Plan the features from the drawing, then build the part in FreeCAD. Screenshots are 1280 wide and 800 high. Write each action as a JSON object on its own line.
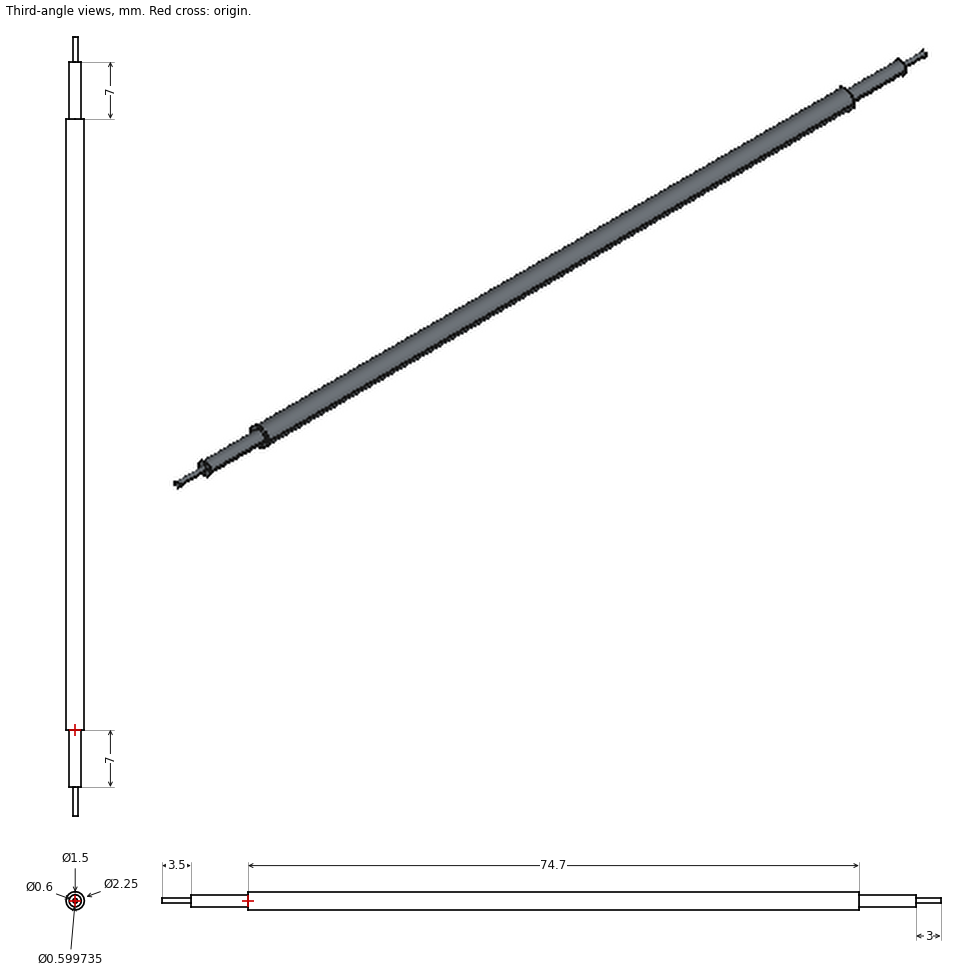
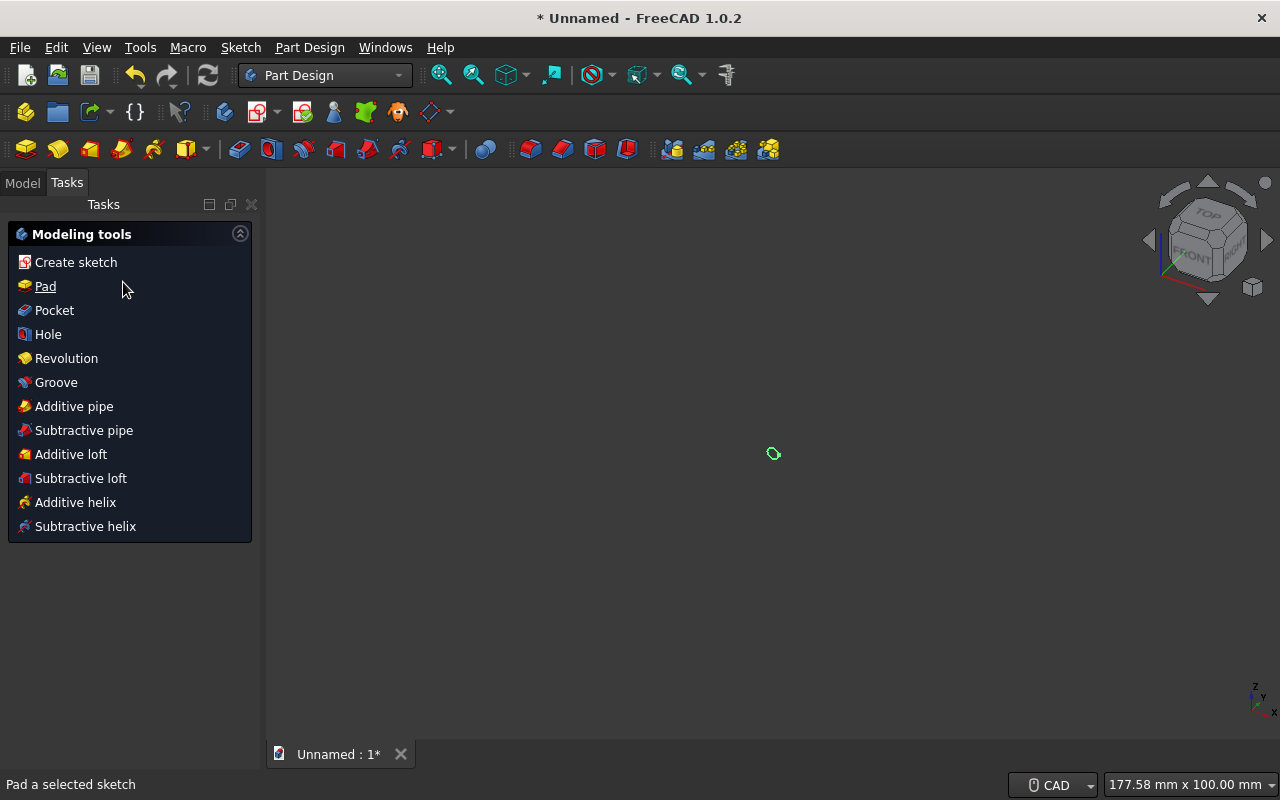
{"action": "left_click", "coordinate": [26, 150]}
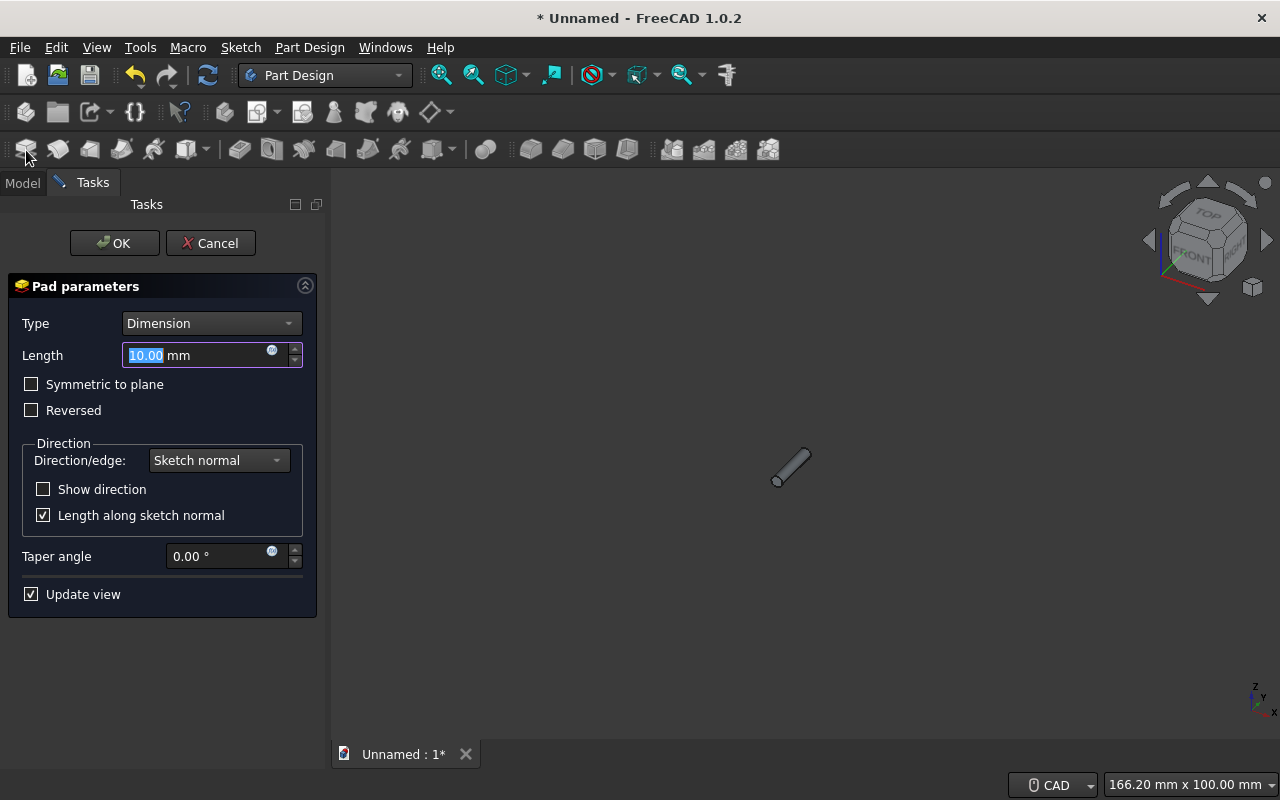
{"action": "type", "text": "74.7"}
{"action": "key", "text": "Tab"}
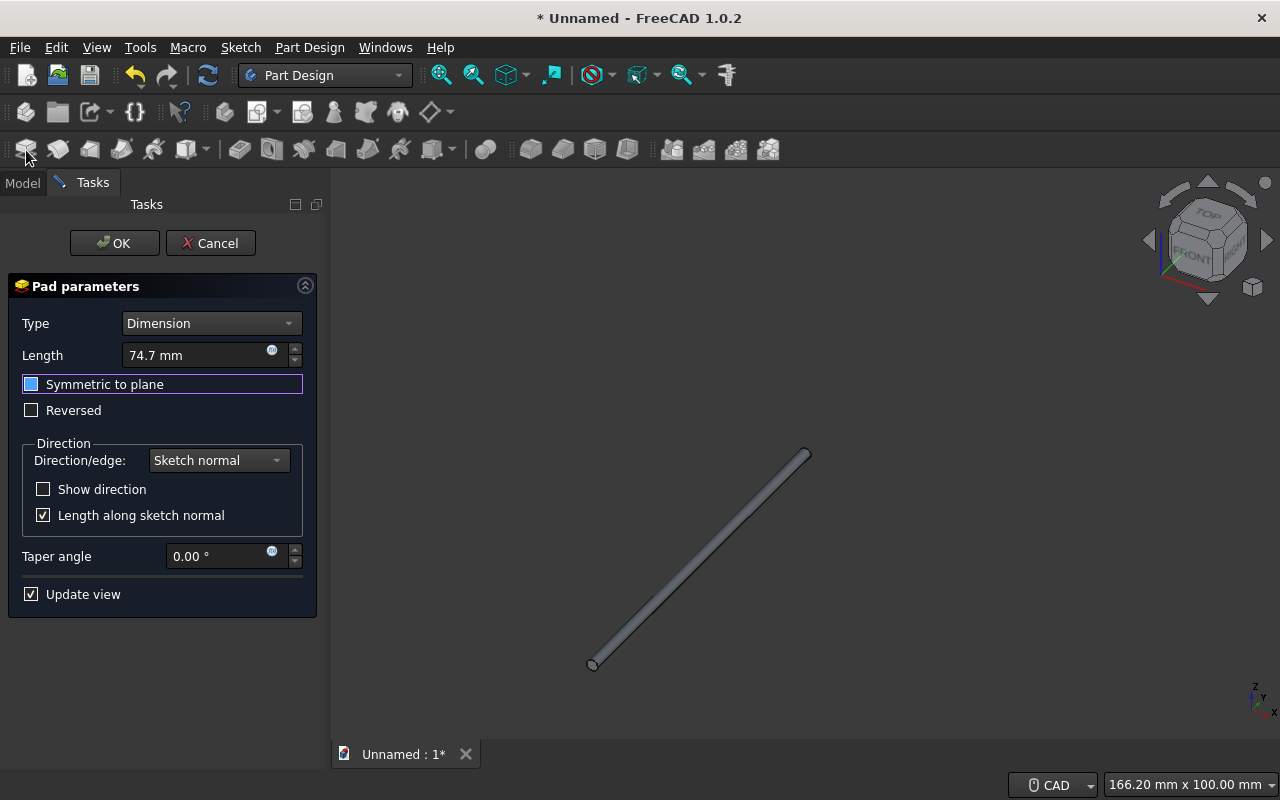
{"action": "left_click", "coordinate": [30, 410]}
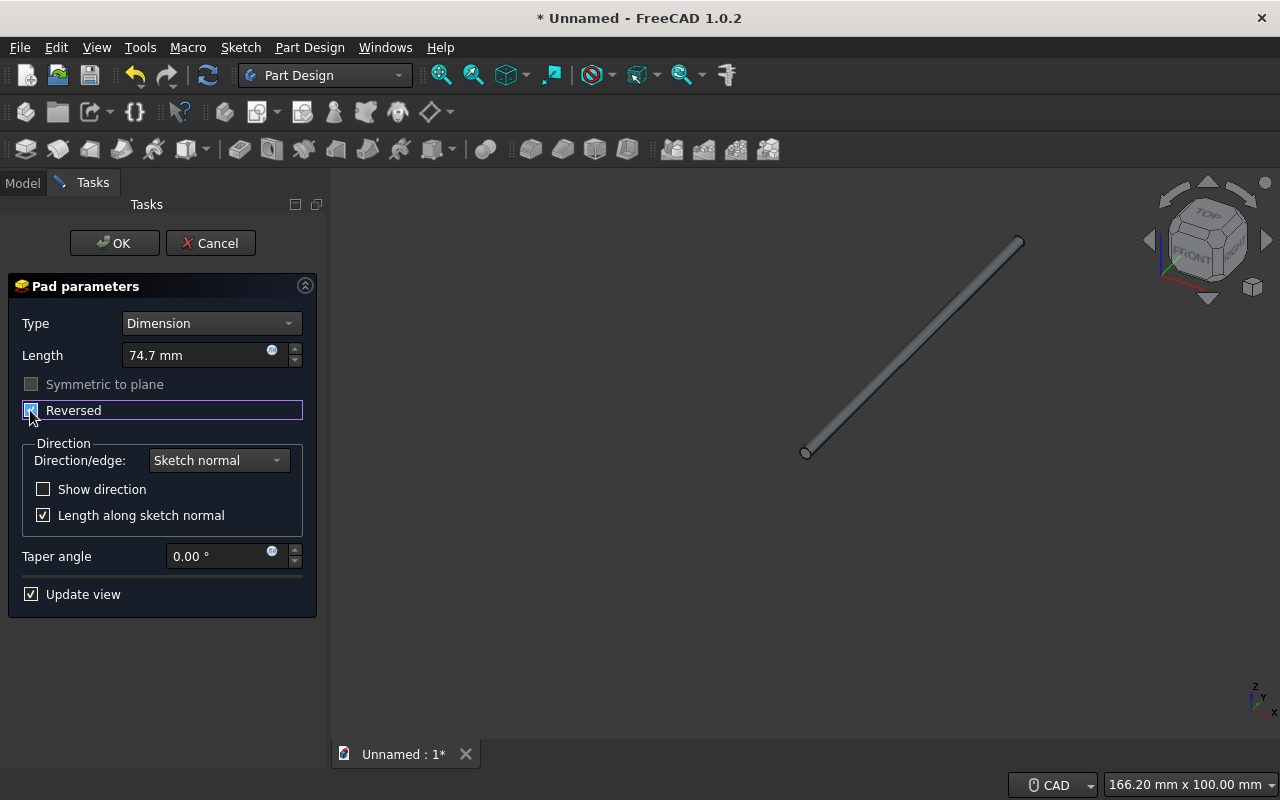
{"action": "left_click", "coordinate": [115, 243]}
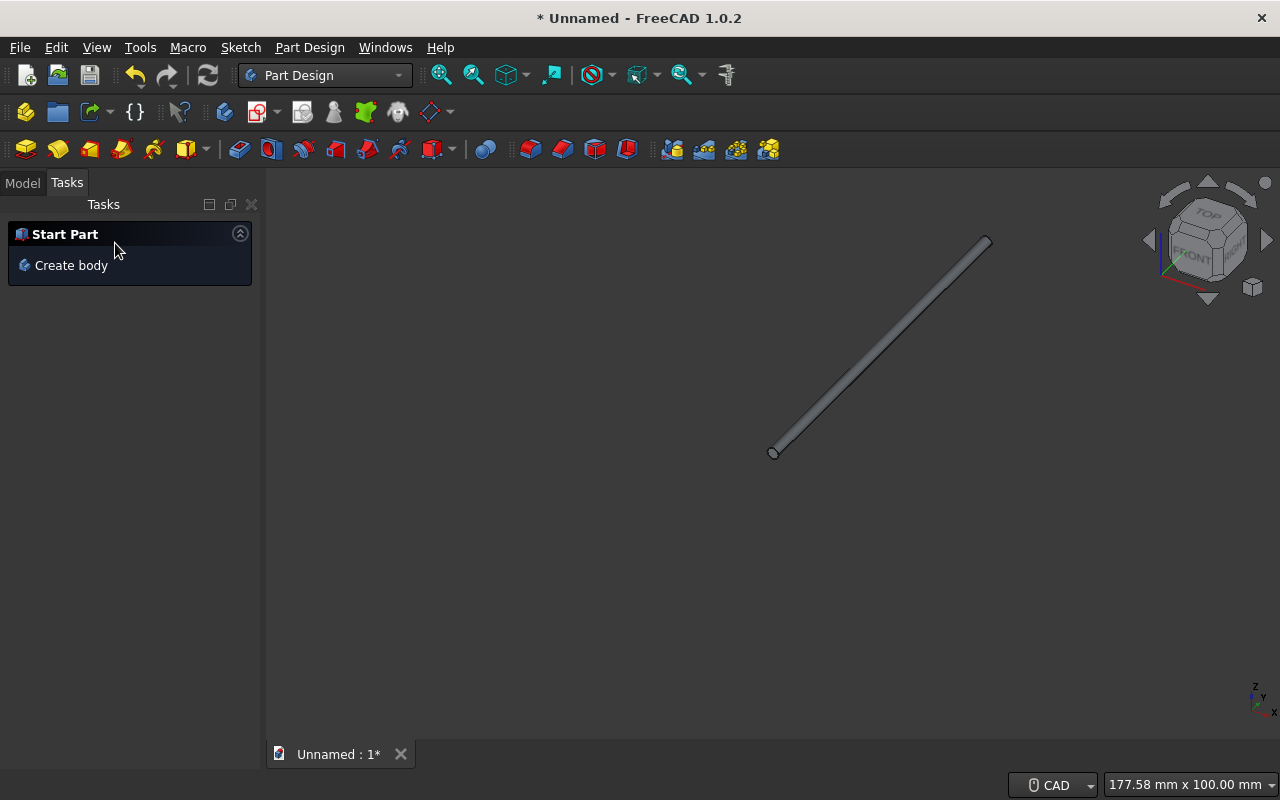
{"action": "left_click", "coordinate": [442, 76]}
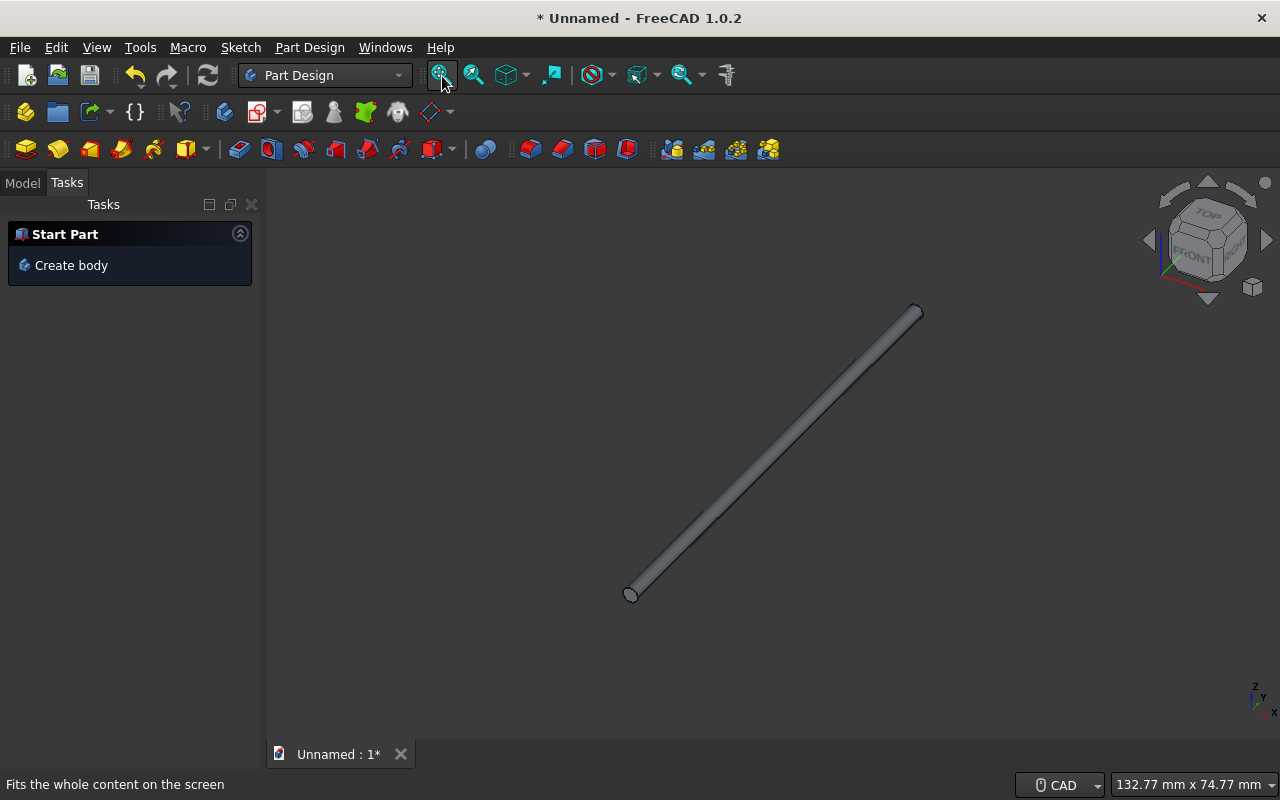
{"action": "left_click", "coordinate": [258, 112]}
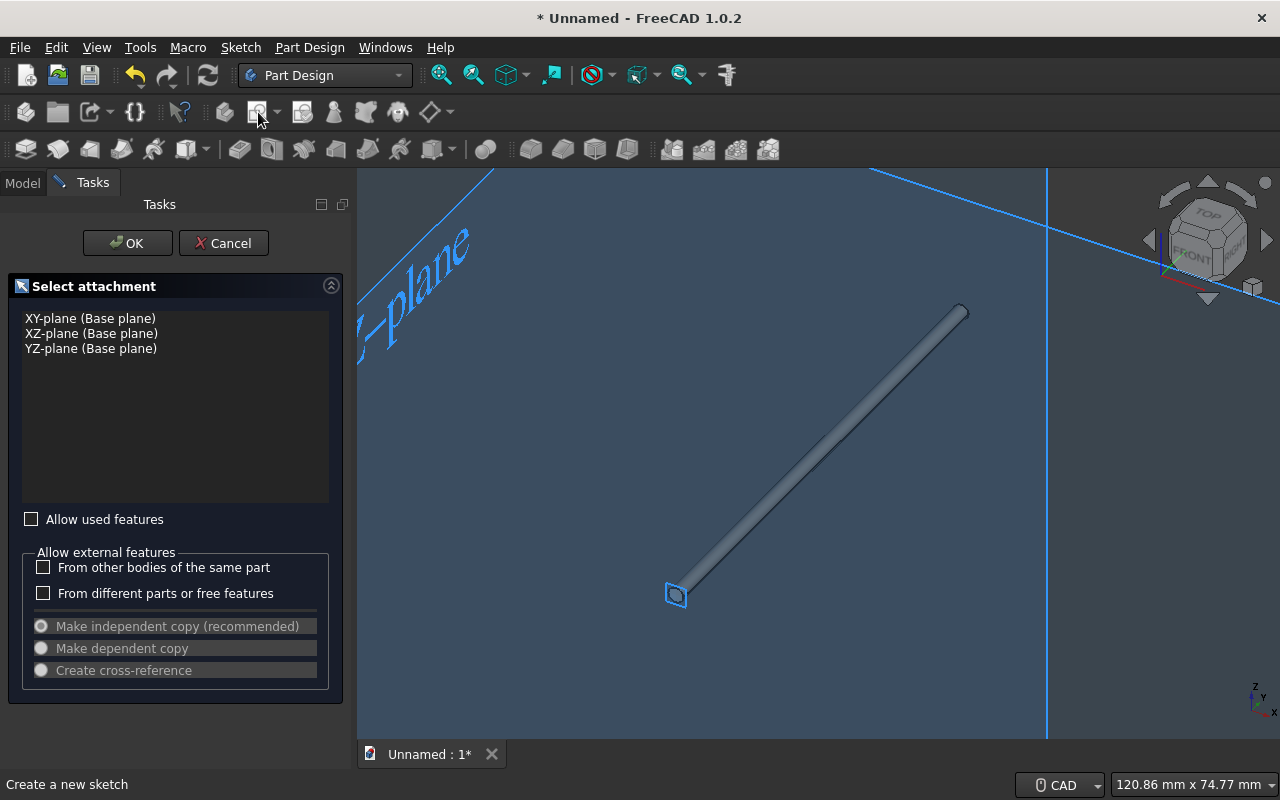
{"action": "left_click", "coordinate": [82, 334]}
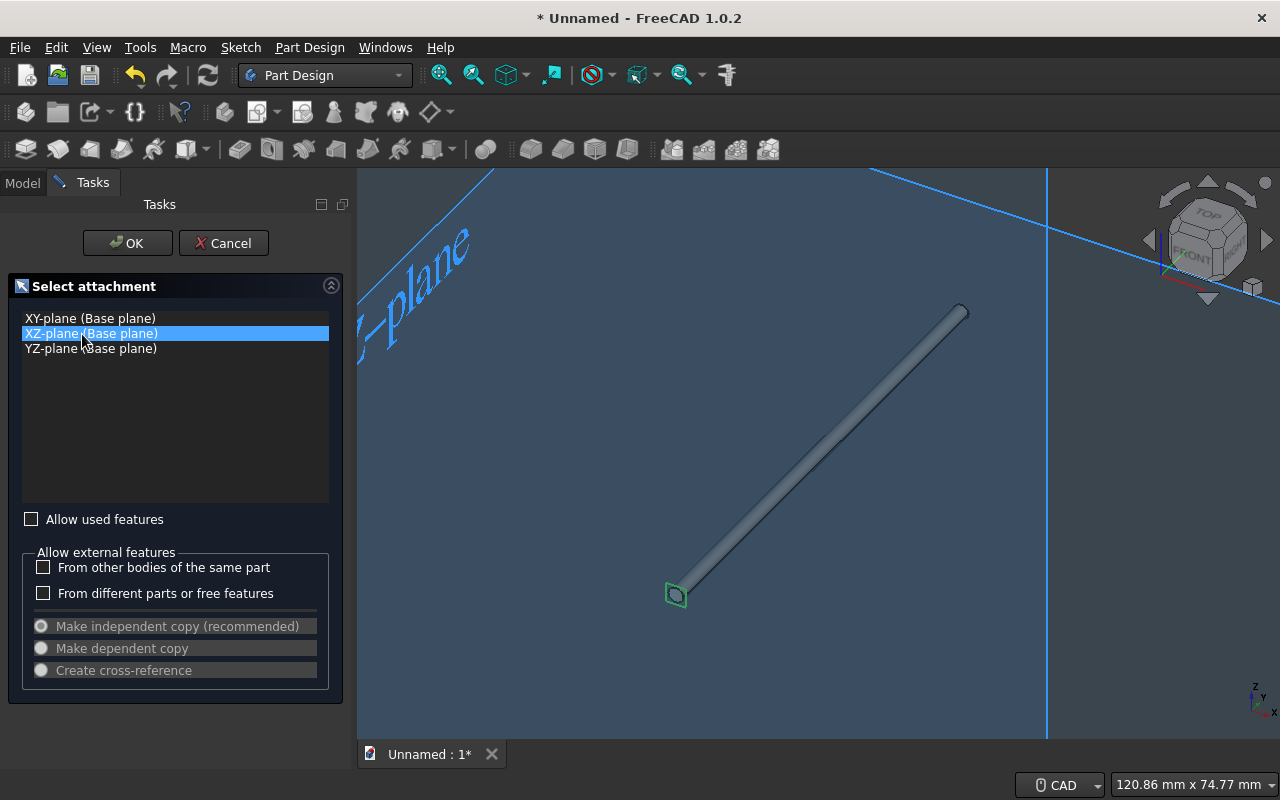
{"action": "left_click", "coordinate": [128, 243]}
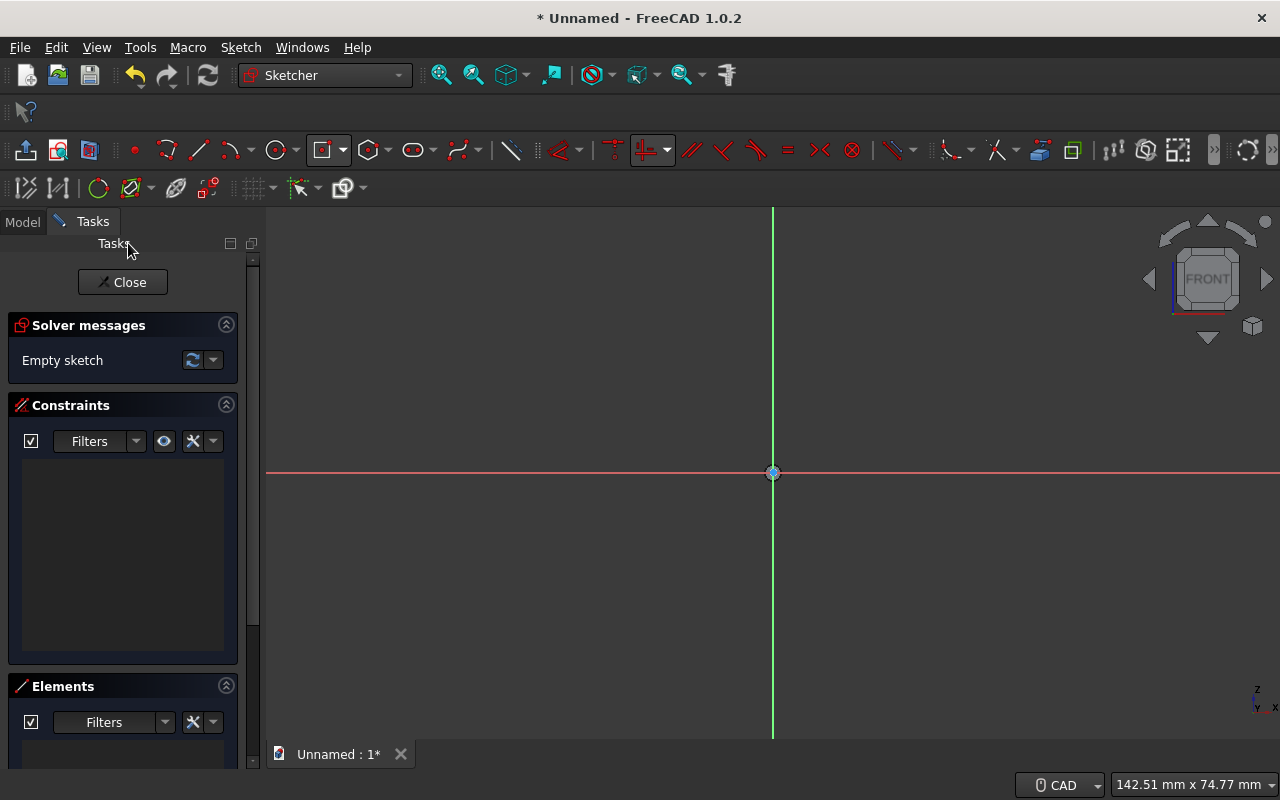
{"action": "scroll", "coordinate": [777, 473], "scroll_direction": "up", "scroll_amount": 15}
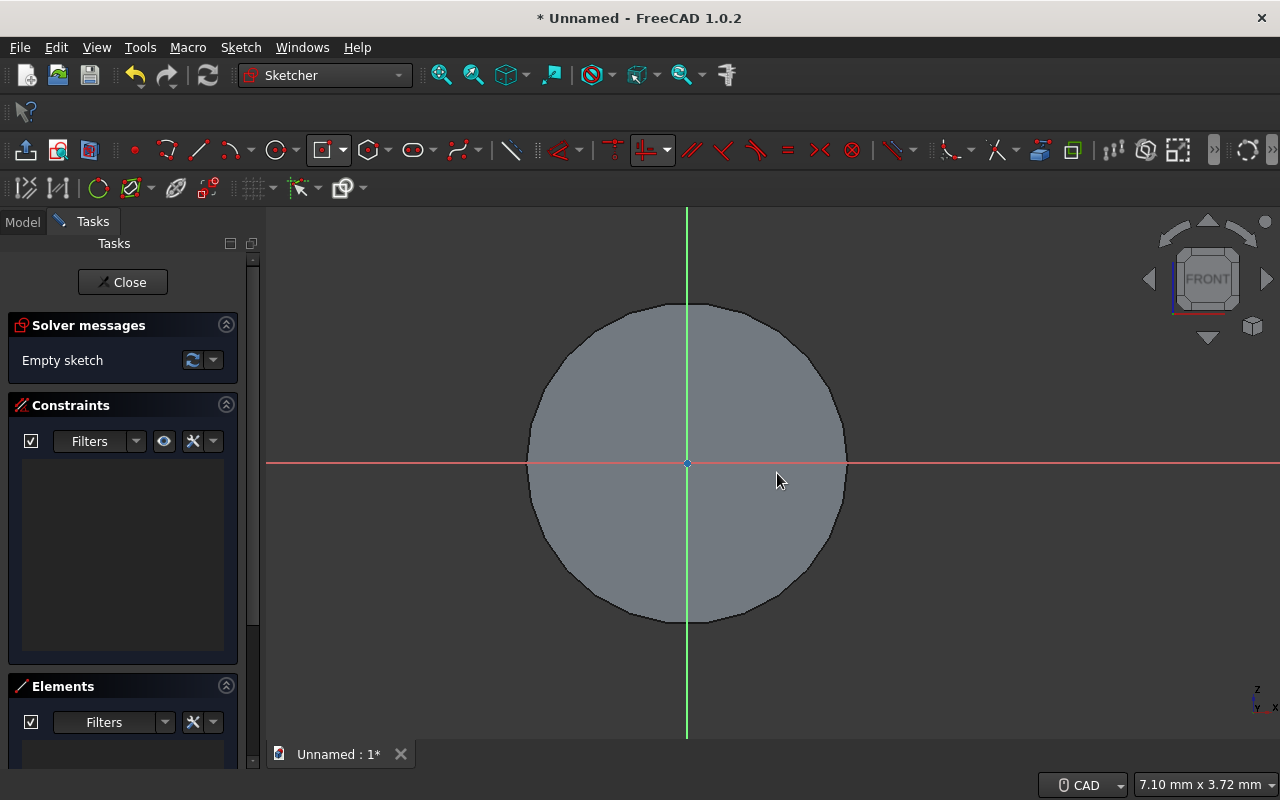
{"action": "scroll", "coordinate": [652, 444], "scroll_direction": "up", "scroll_amount": 2}